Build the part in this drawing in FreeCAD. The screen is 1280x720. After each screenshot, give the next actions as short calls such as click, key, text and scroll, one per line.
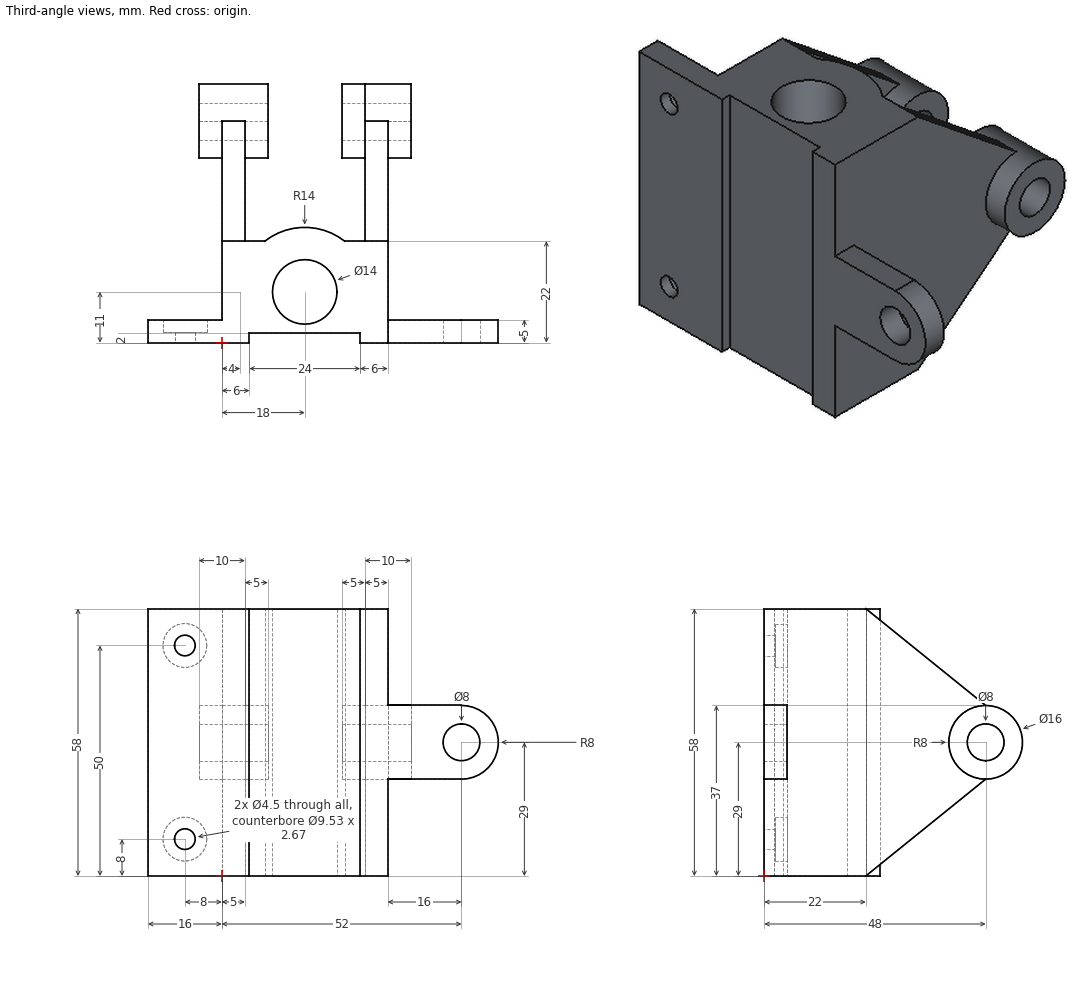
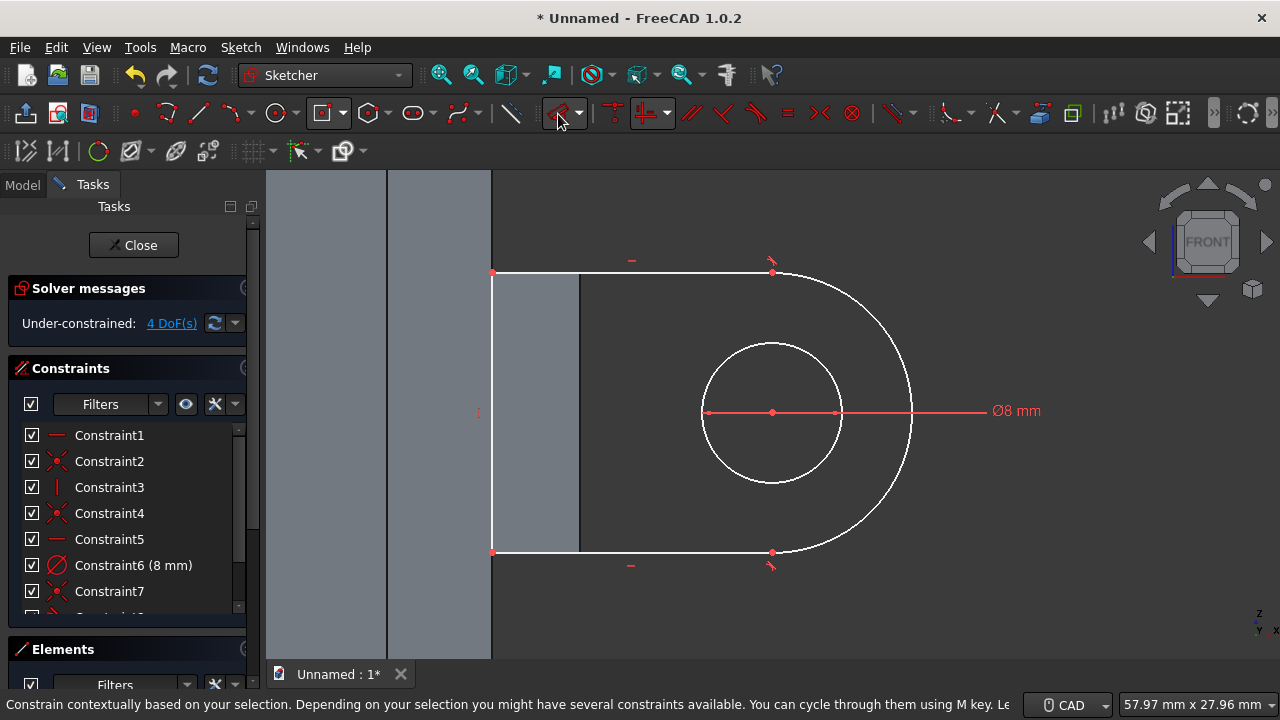
click(885, 495)
click(911, 514)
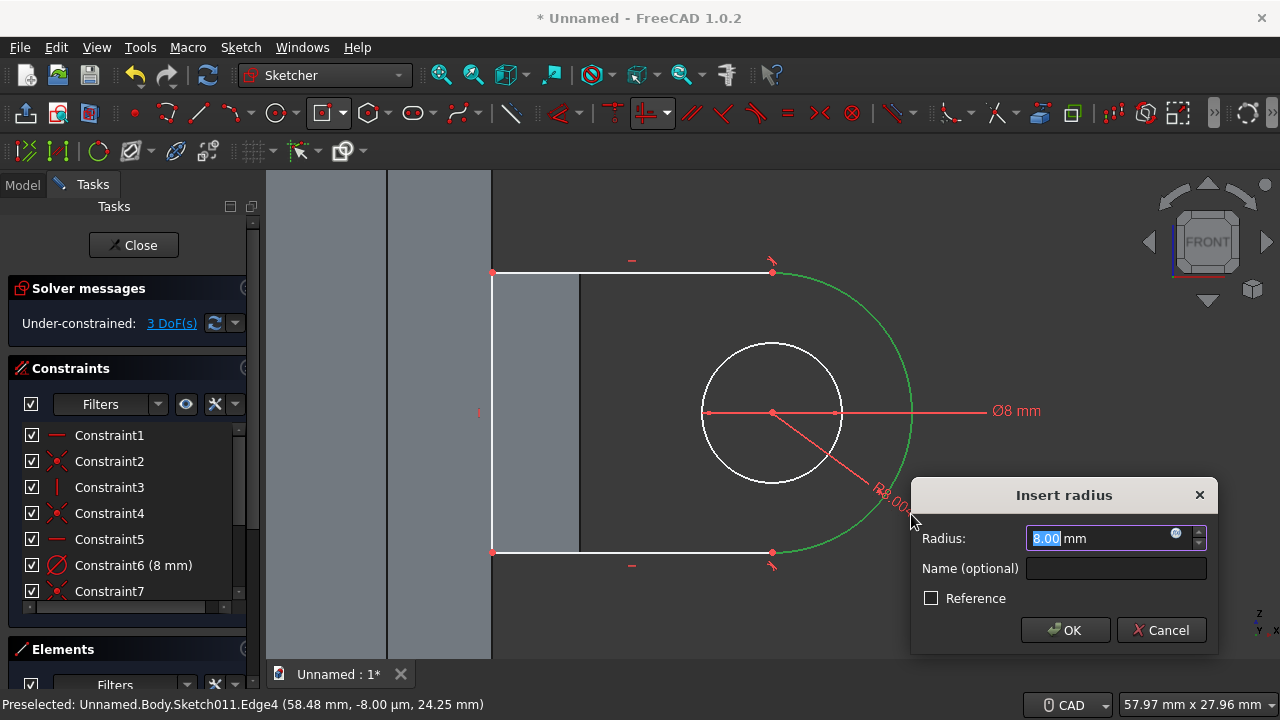
text(8)
key(Return)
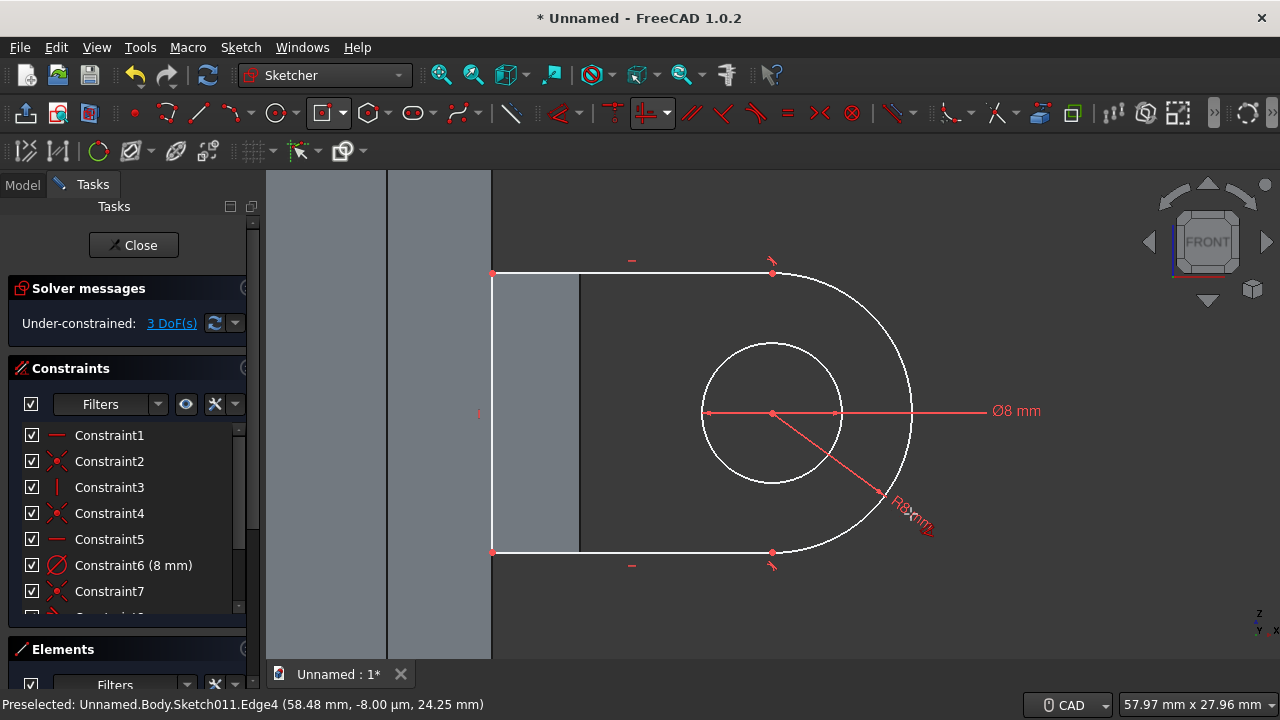
click(688, 553)
click(632, 587)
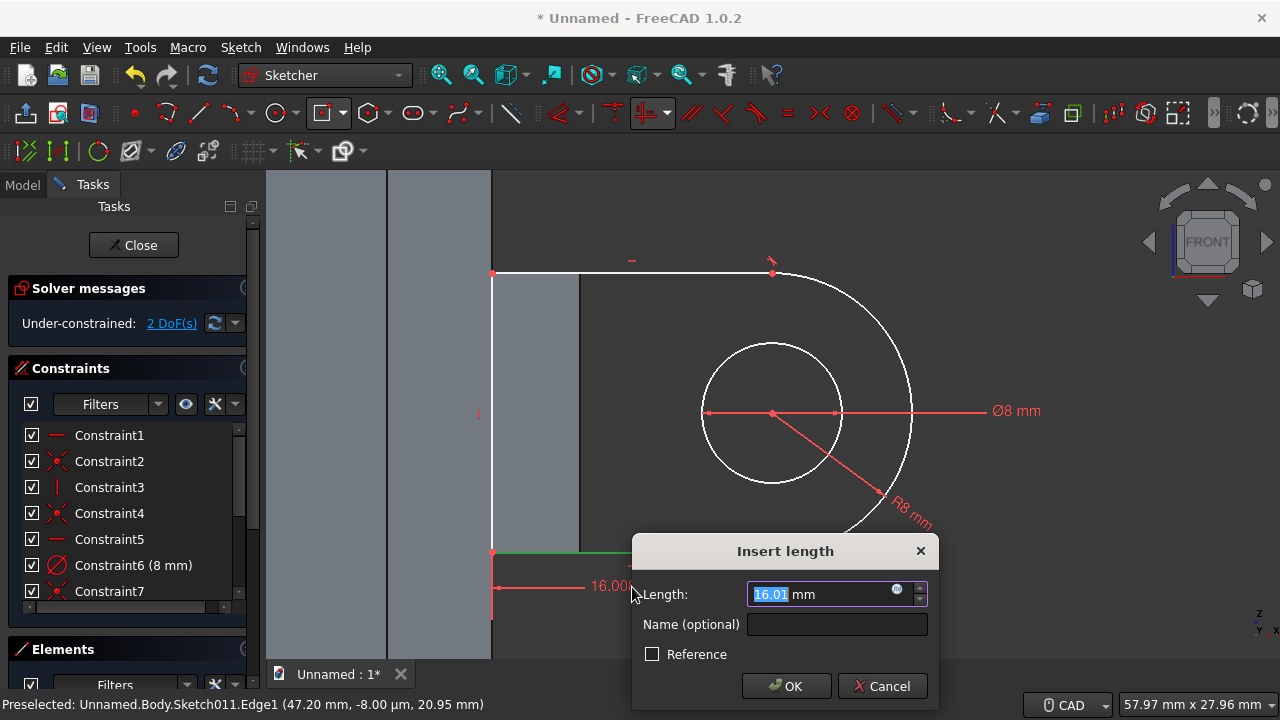
text(16)
key(Return)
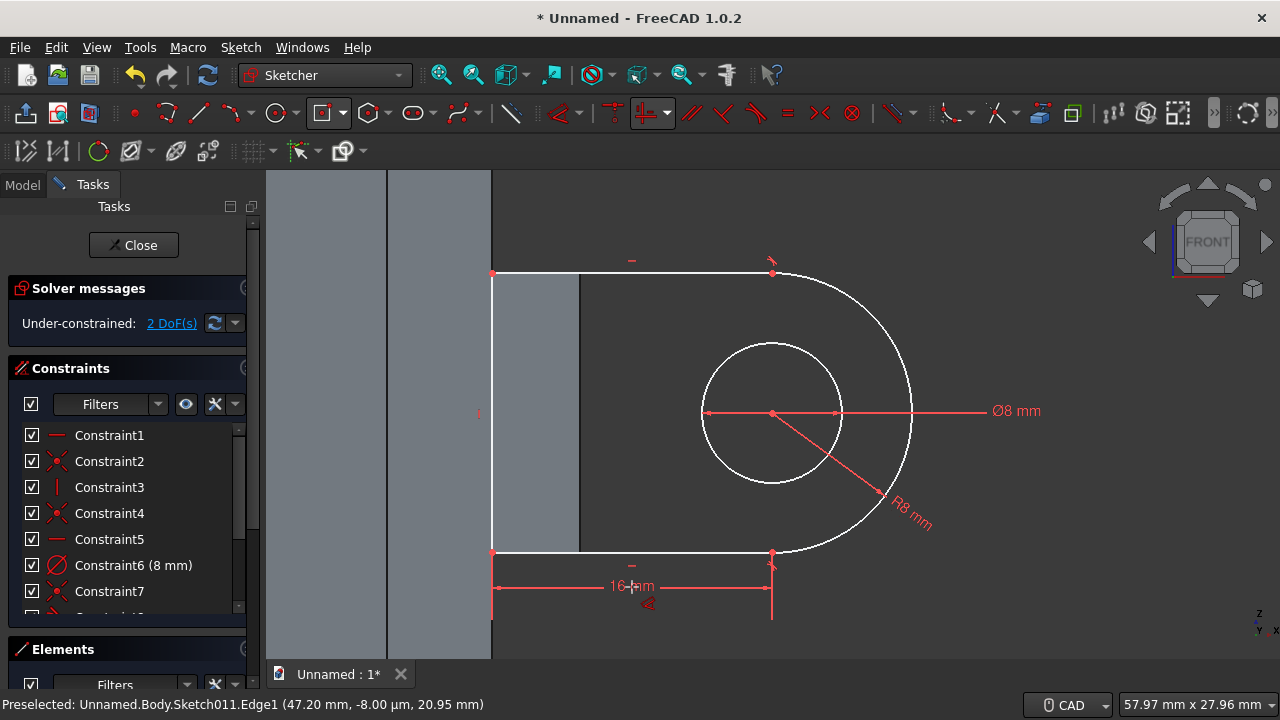
click(772, 413)
click(533, 379)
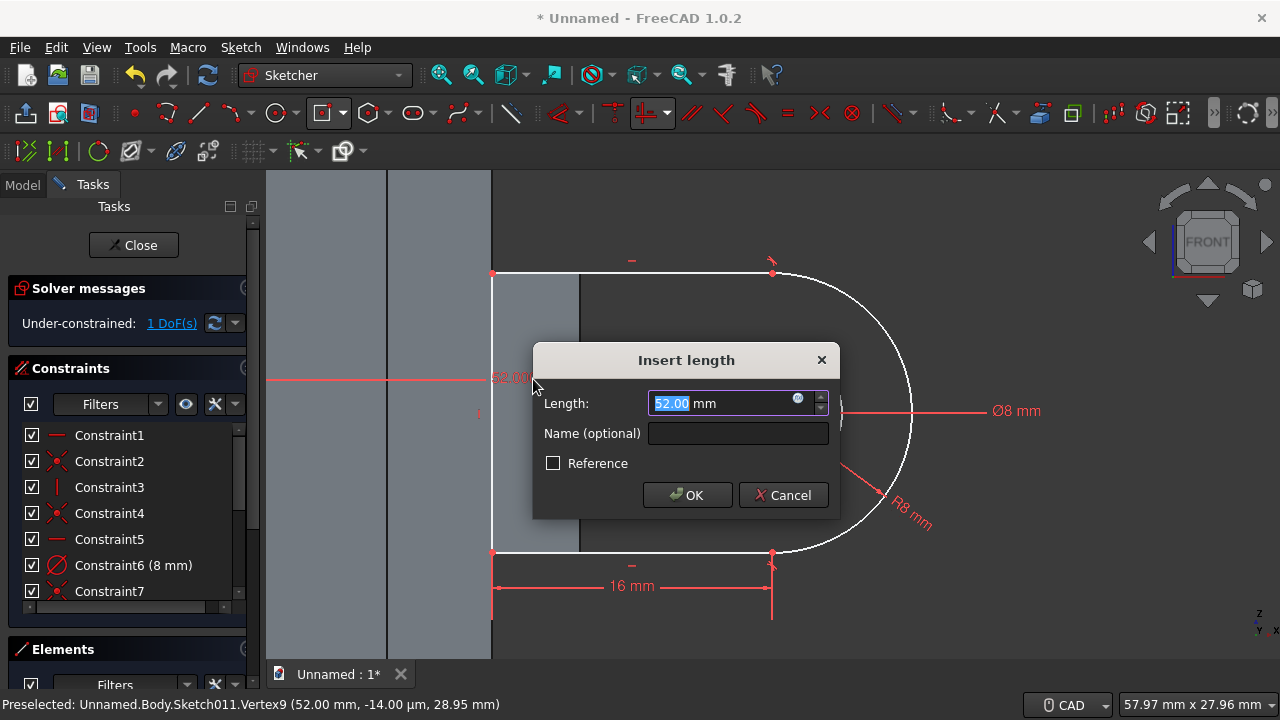
text(52)
key(Return)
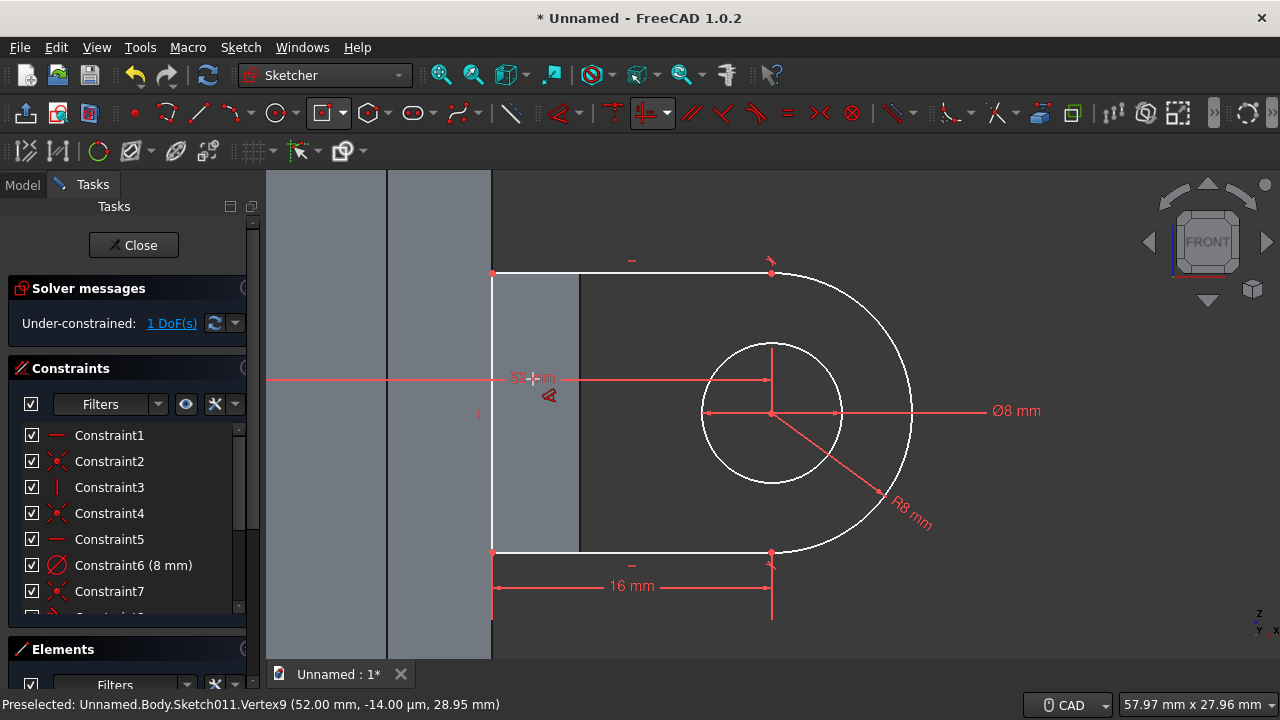
click(772, 413)
click(806, 522)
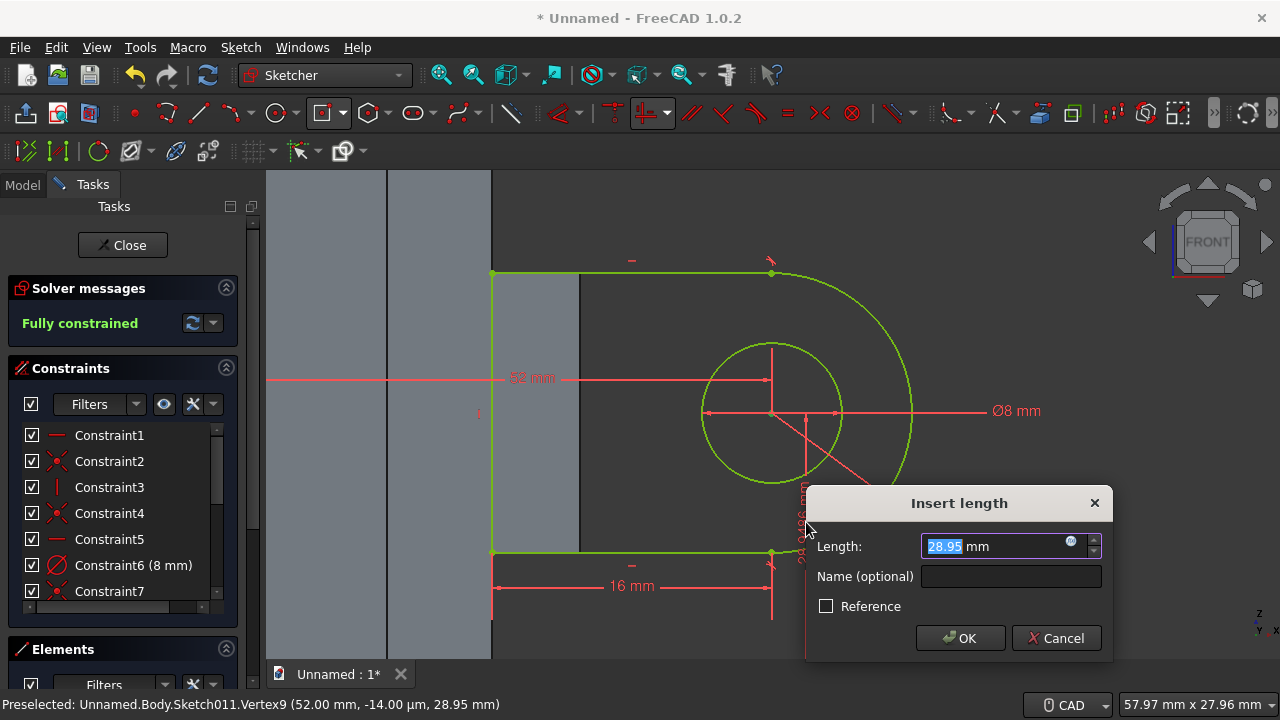
text(29)
key(Return)
key(Escape)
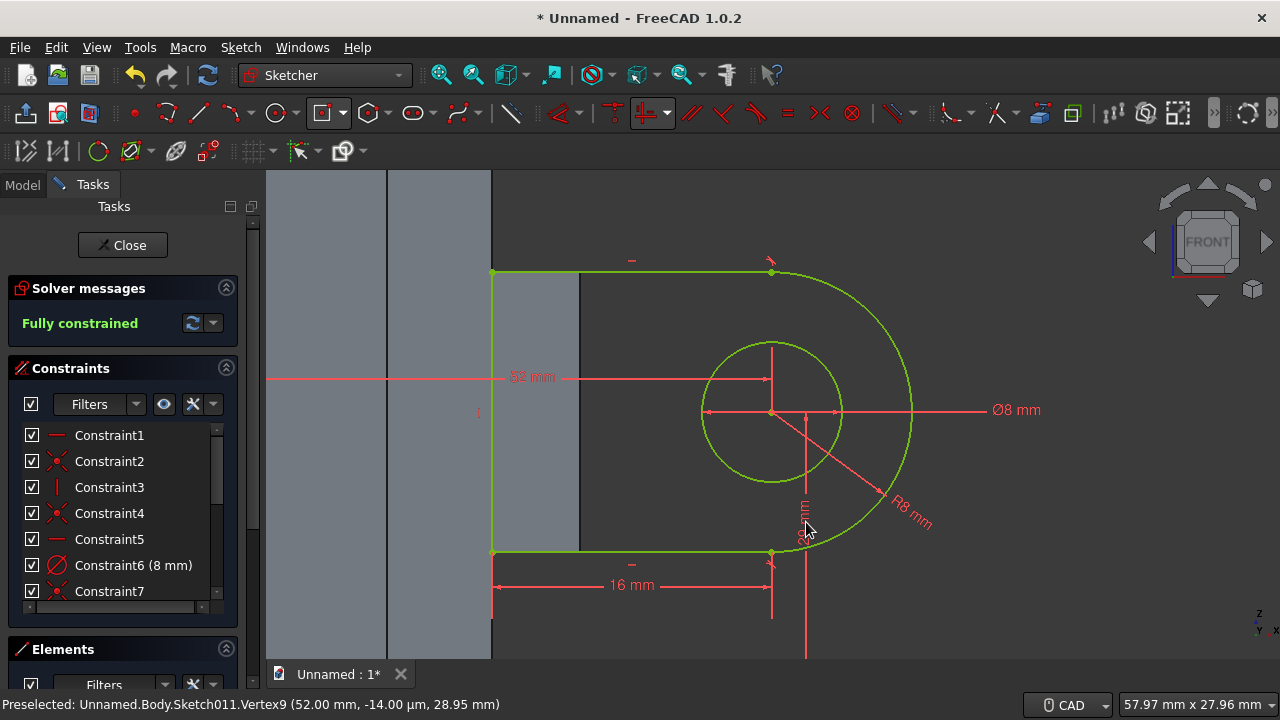
click(123, 245)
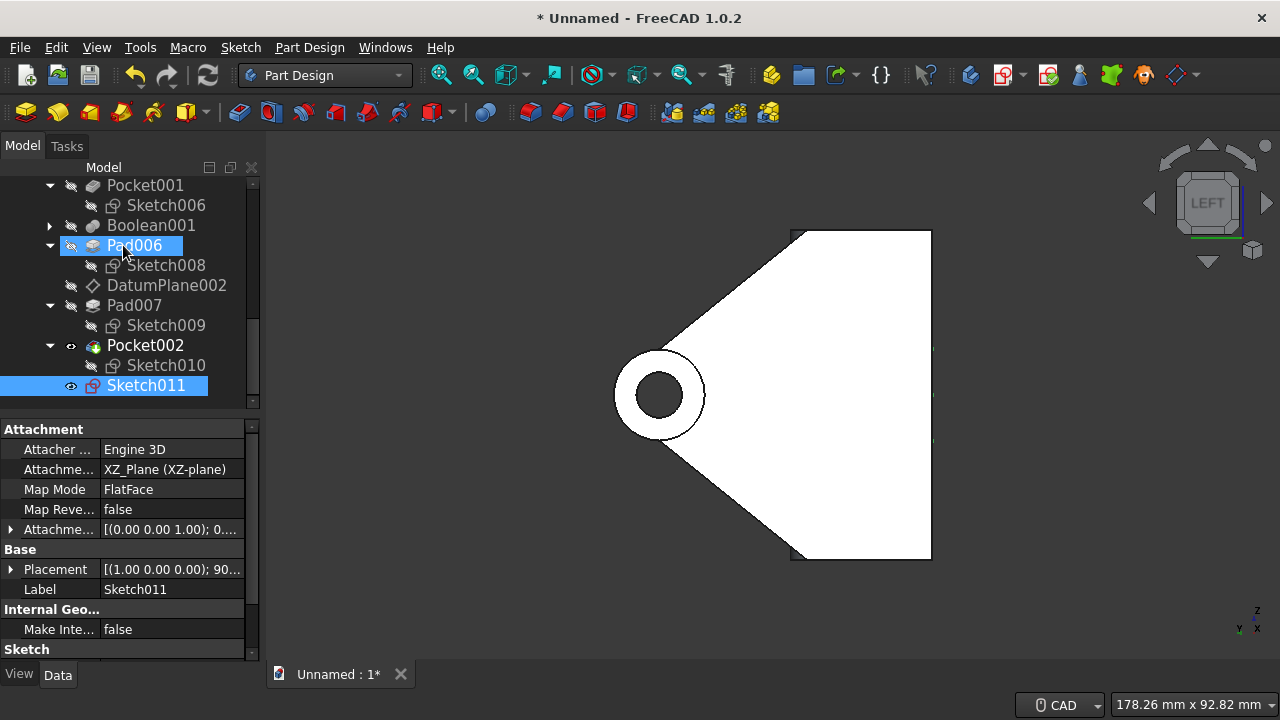
click(26, 112)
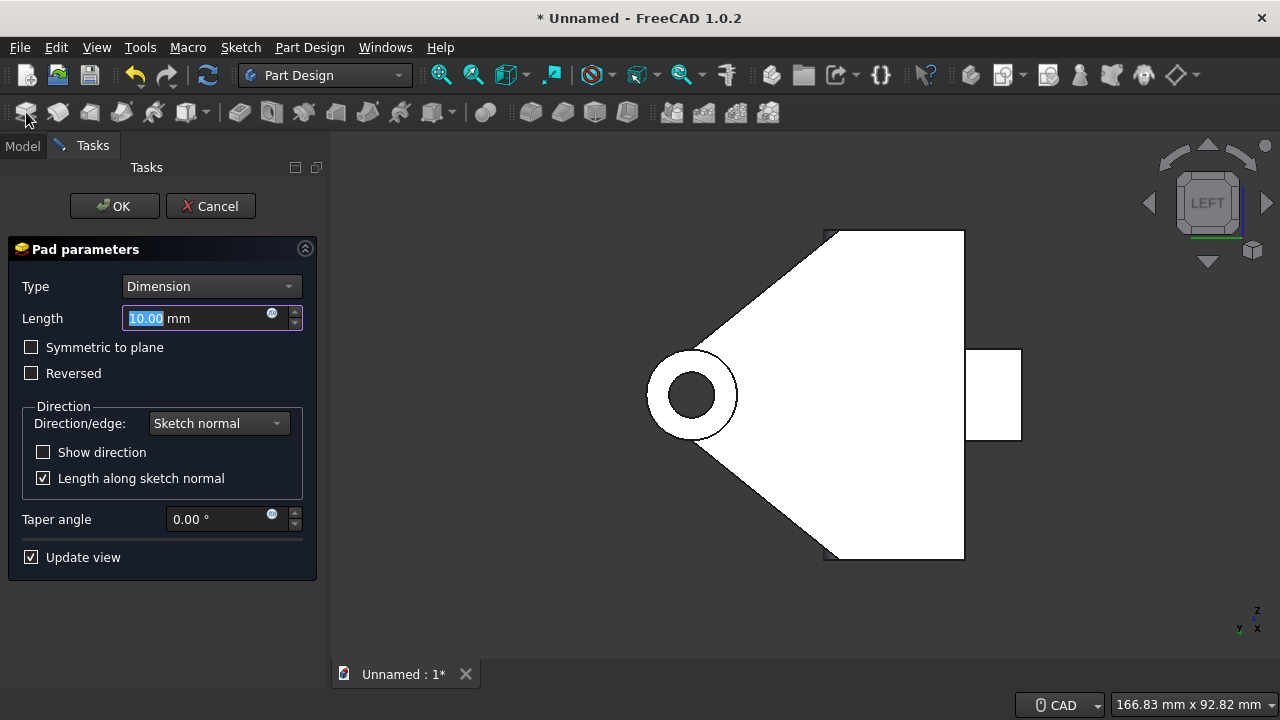
text(5)
key(Tab)